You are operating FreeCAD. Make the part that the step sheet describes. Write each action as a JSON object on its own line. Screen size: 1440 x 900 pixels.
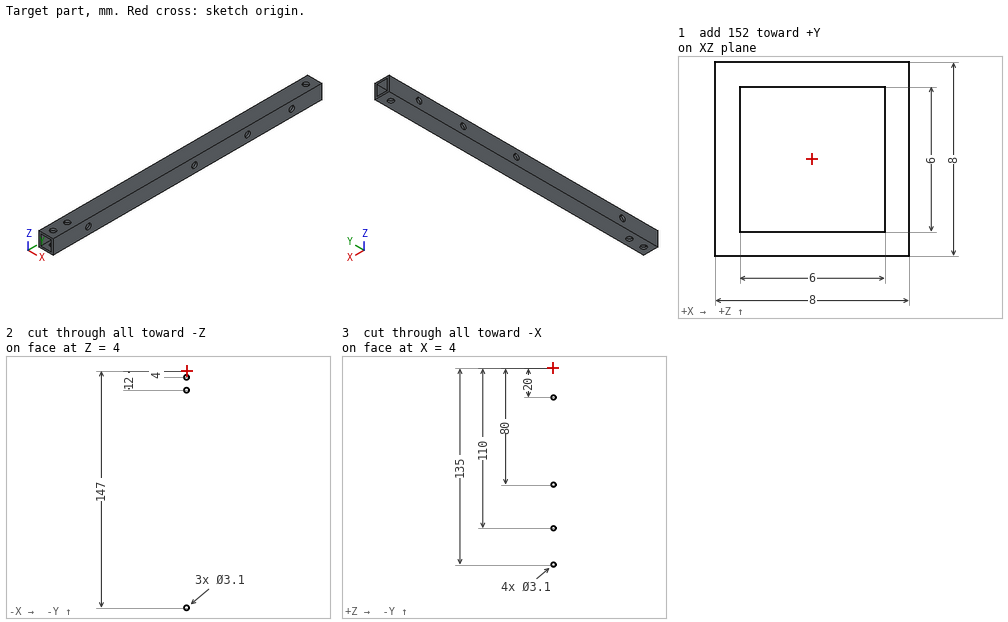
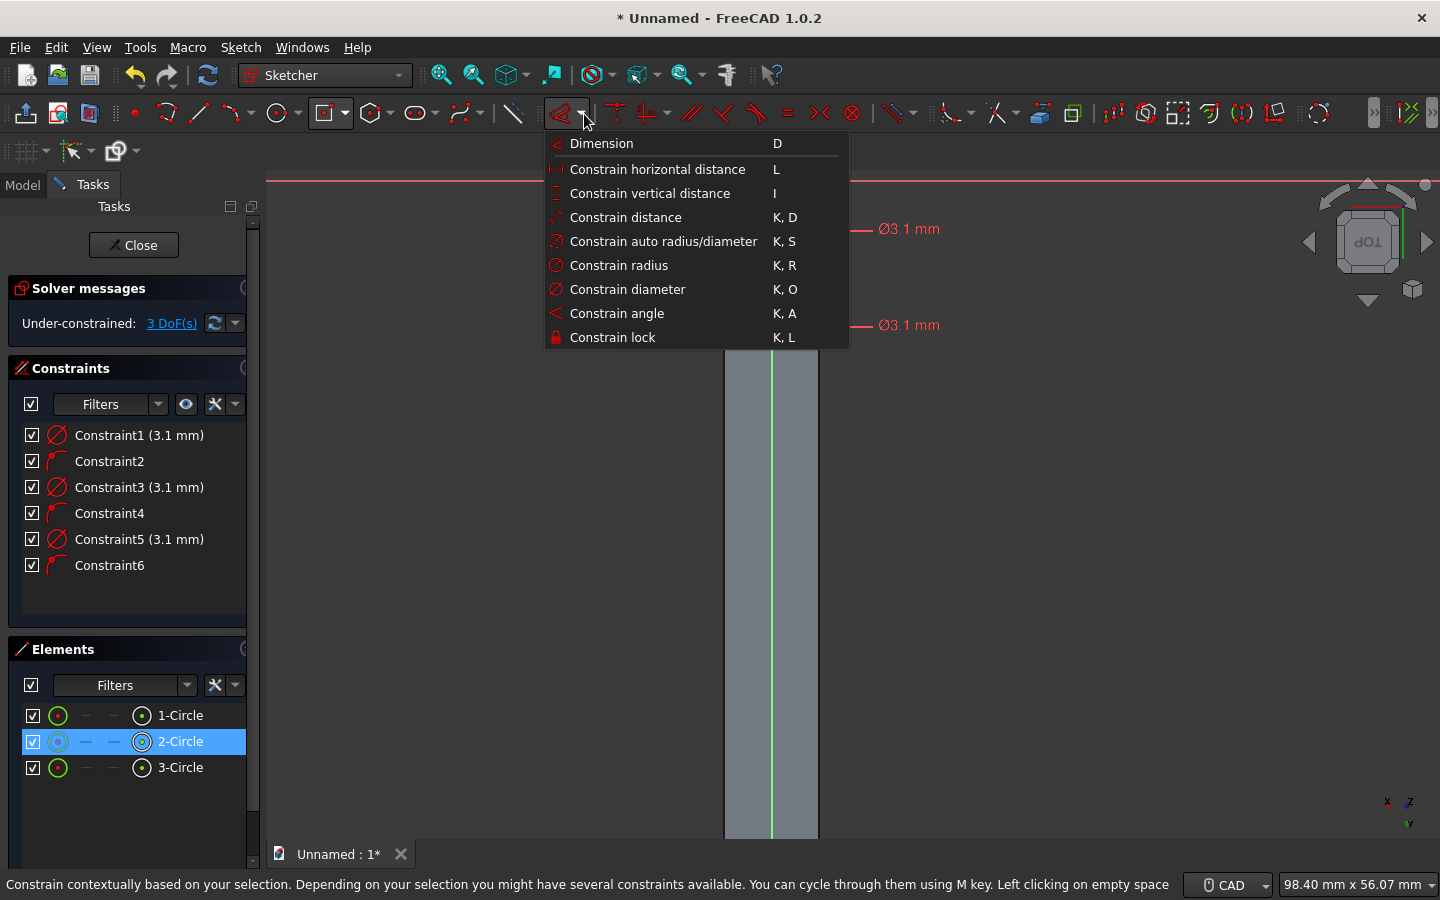
{"action": "left_click", "coordinate": [697, 193]}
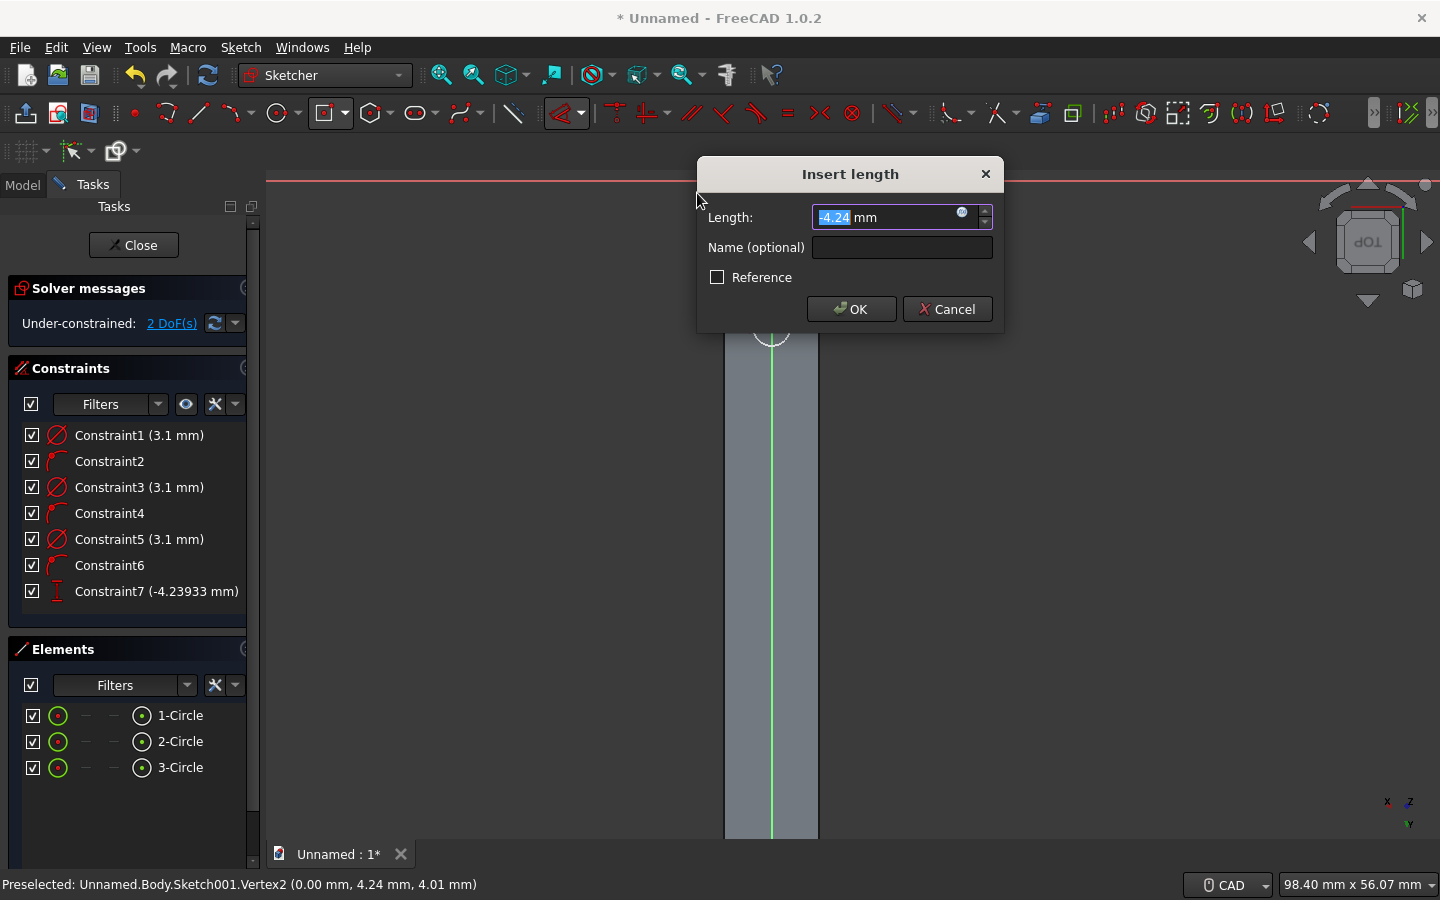
{"action": "type", "text": "-4"}
{"action": "key", "text": "Return"}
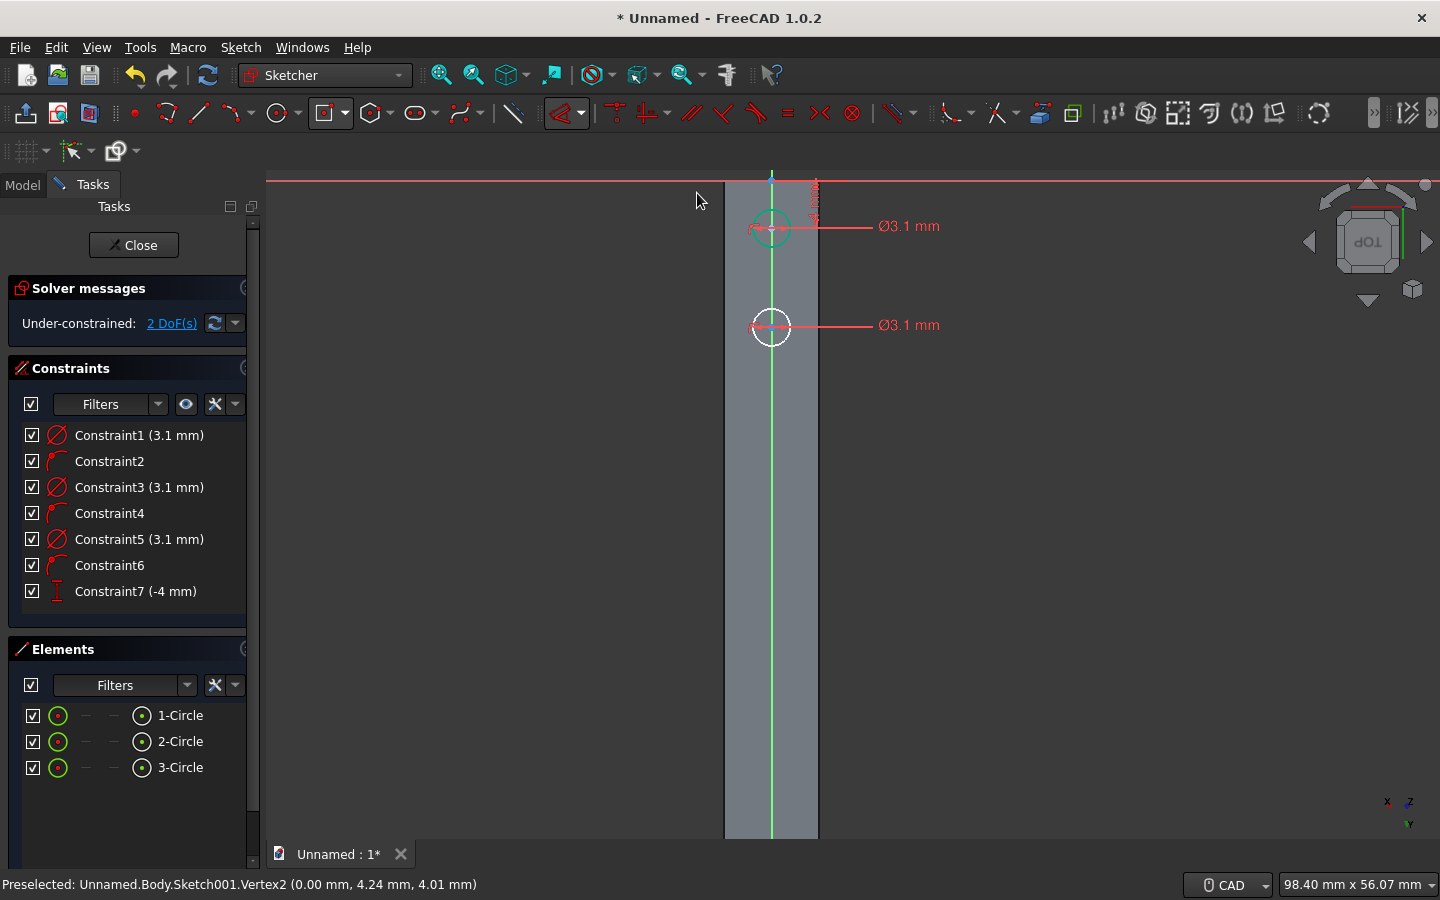
{"action": "scroll", "coordinate": [789, 320], "scroll_direction": "down", "scroll_amount": 7}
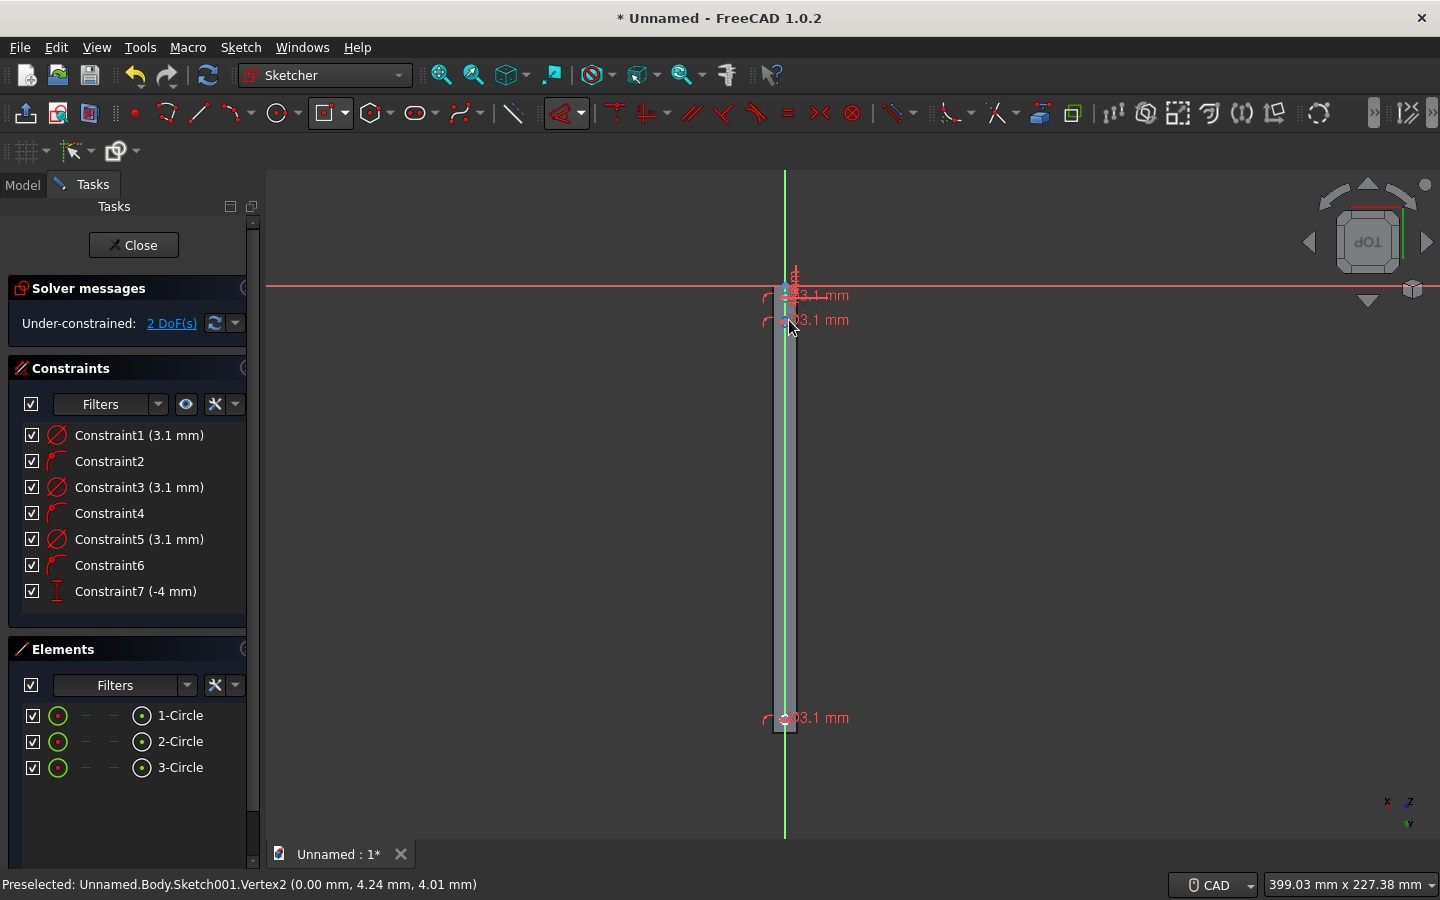
{"action": "left_click", "coordinate": [785, 322]}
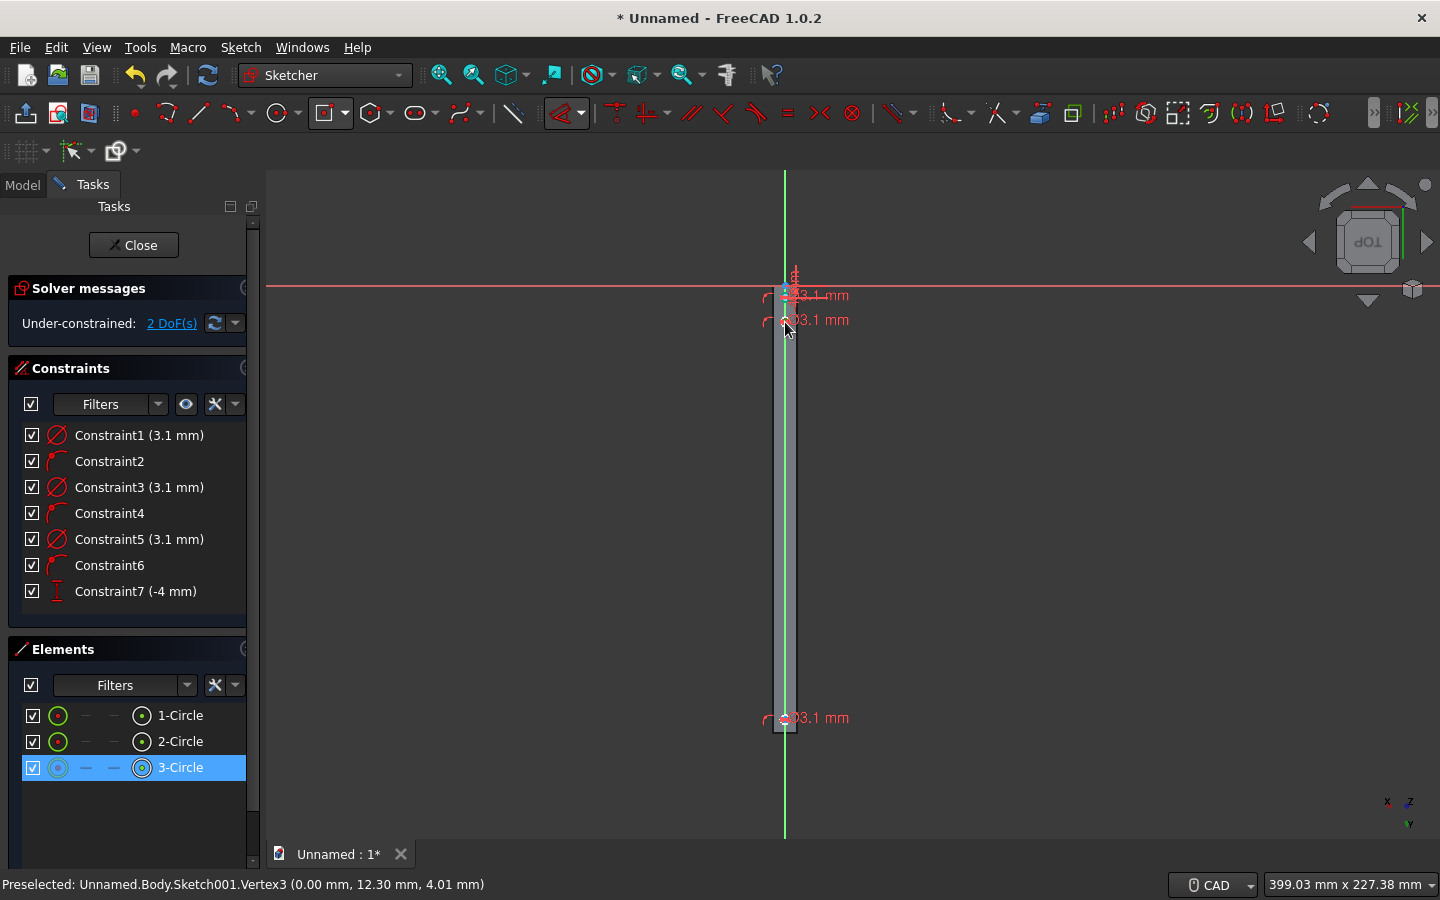
{"action": "key", "text": "i"}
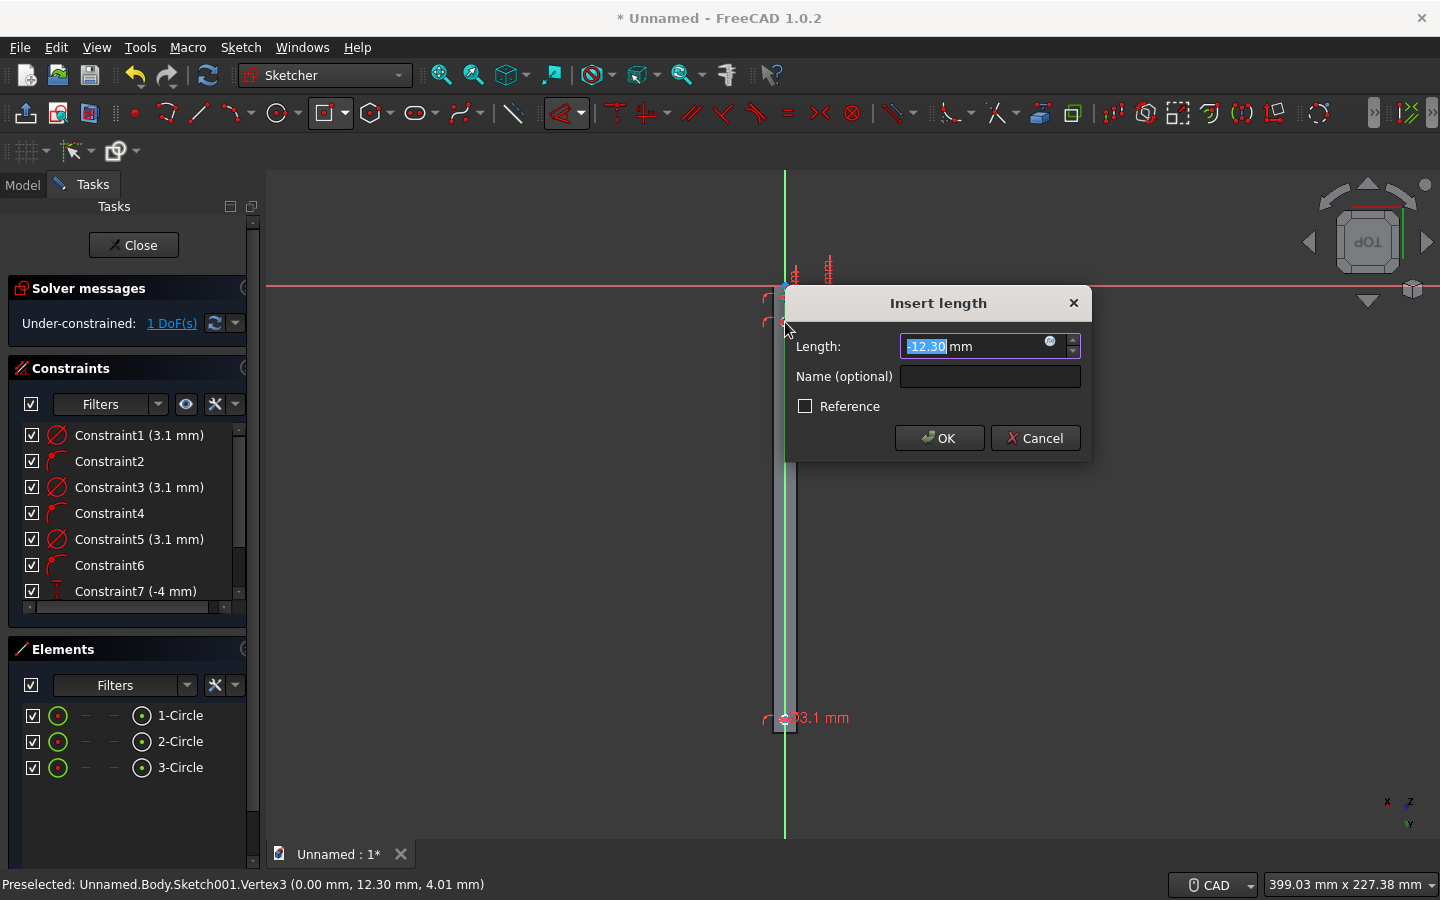
{"action": "type", "text": "-12"}
{"action": "key", "text": "Return"}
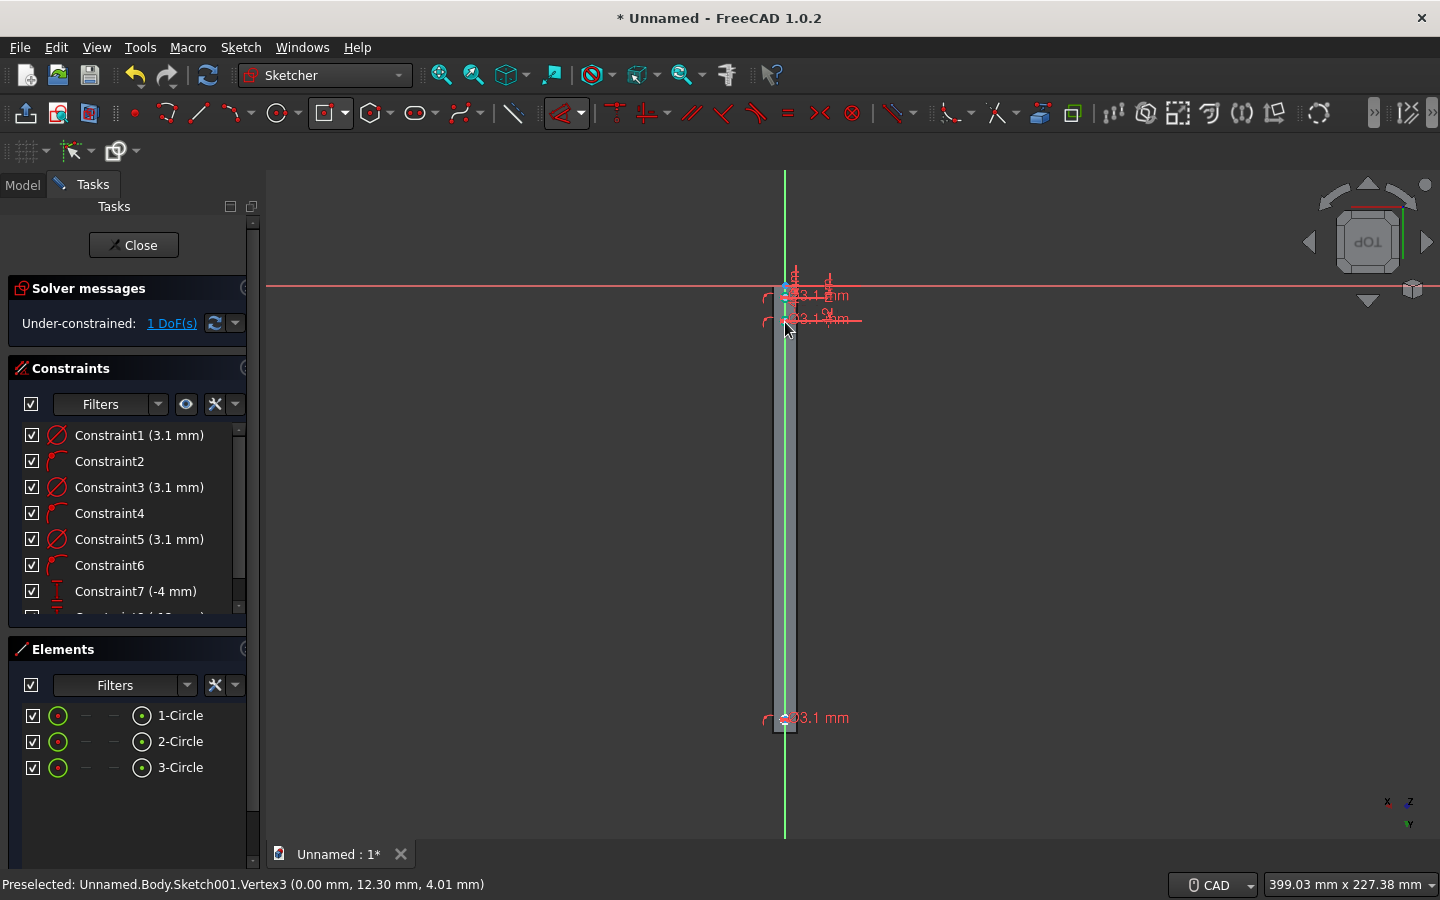
{"action": "left_click", "coordinate": [785, 720]}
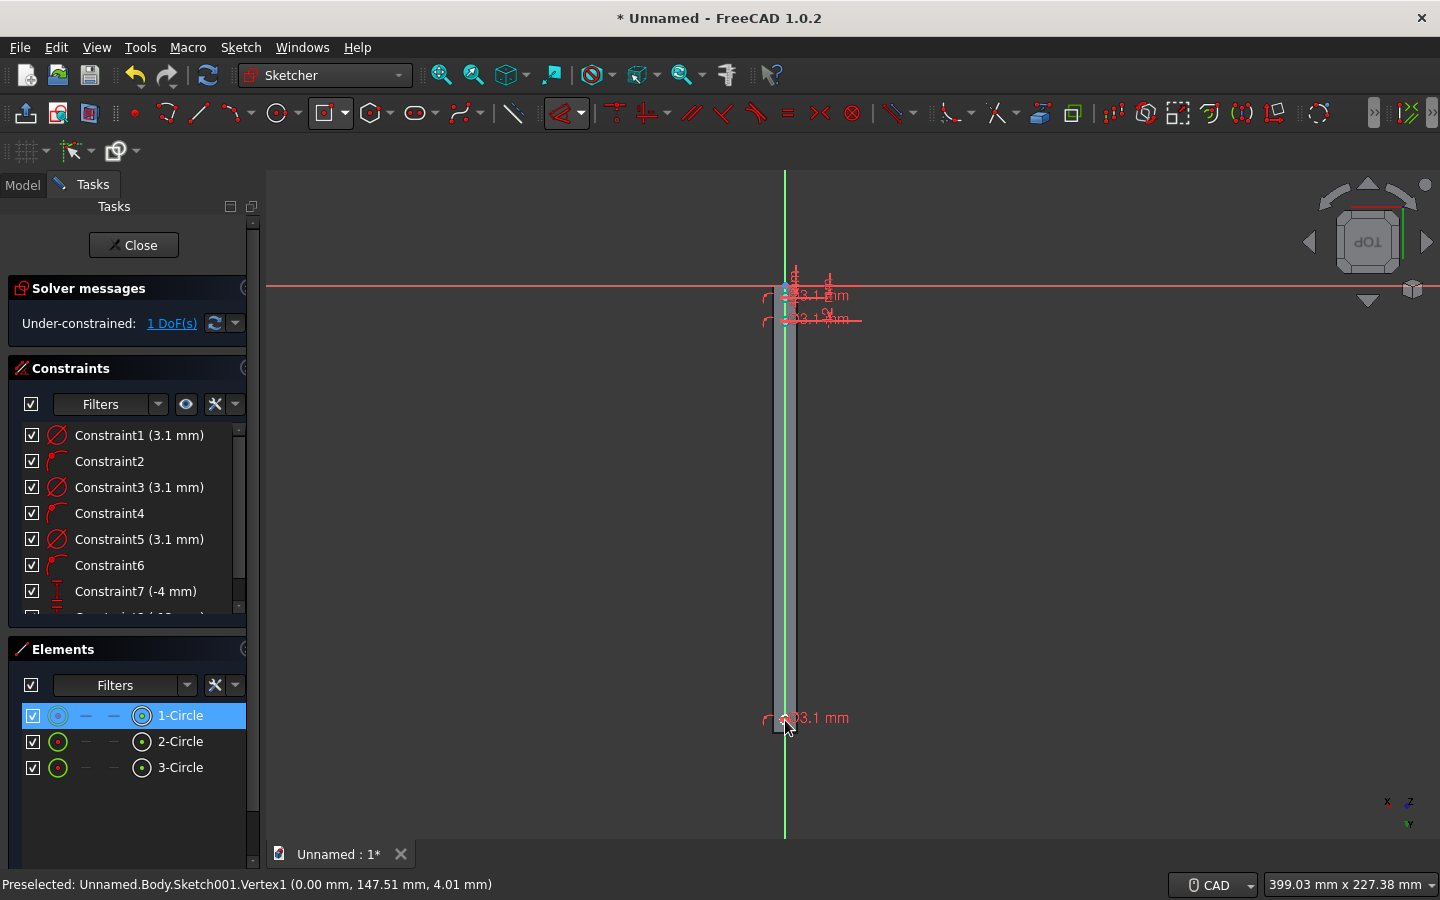
{"action": "left_click", "coordinate": [584, 114]}